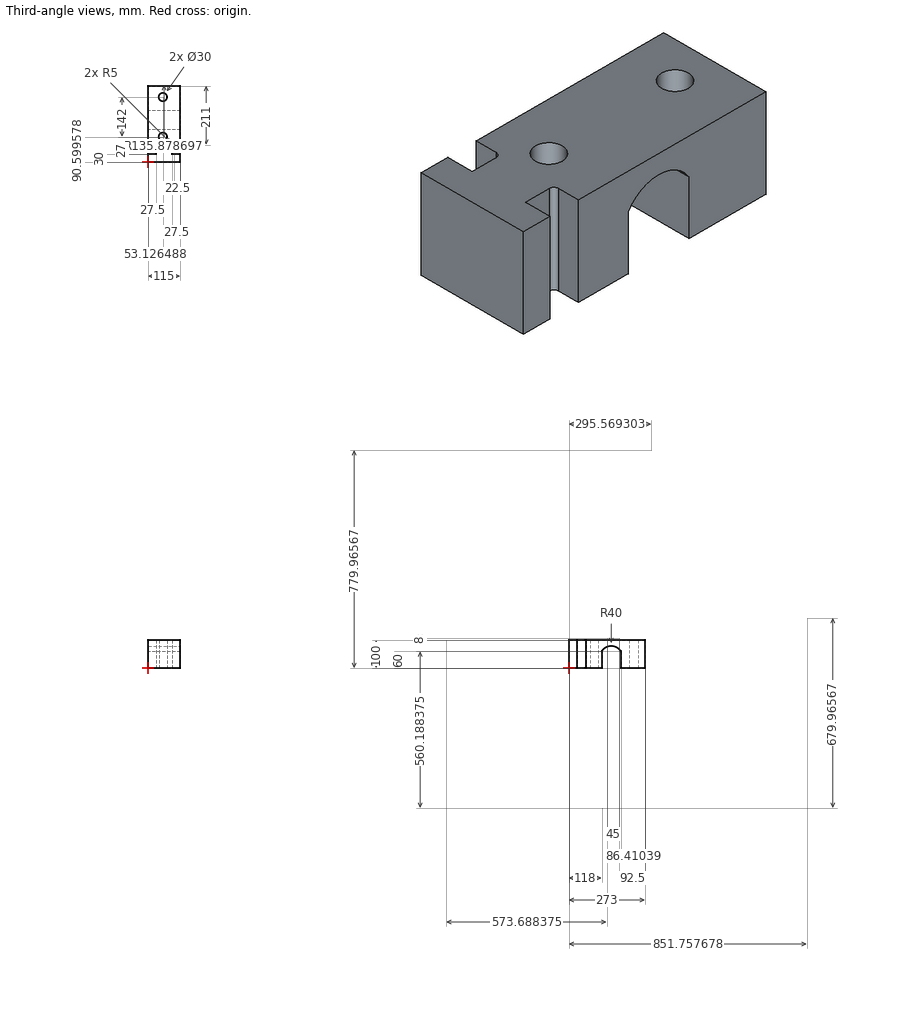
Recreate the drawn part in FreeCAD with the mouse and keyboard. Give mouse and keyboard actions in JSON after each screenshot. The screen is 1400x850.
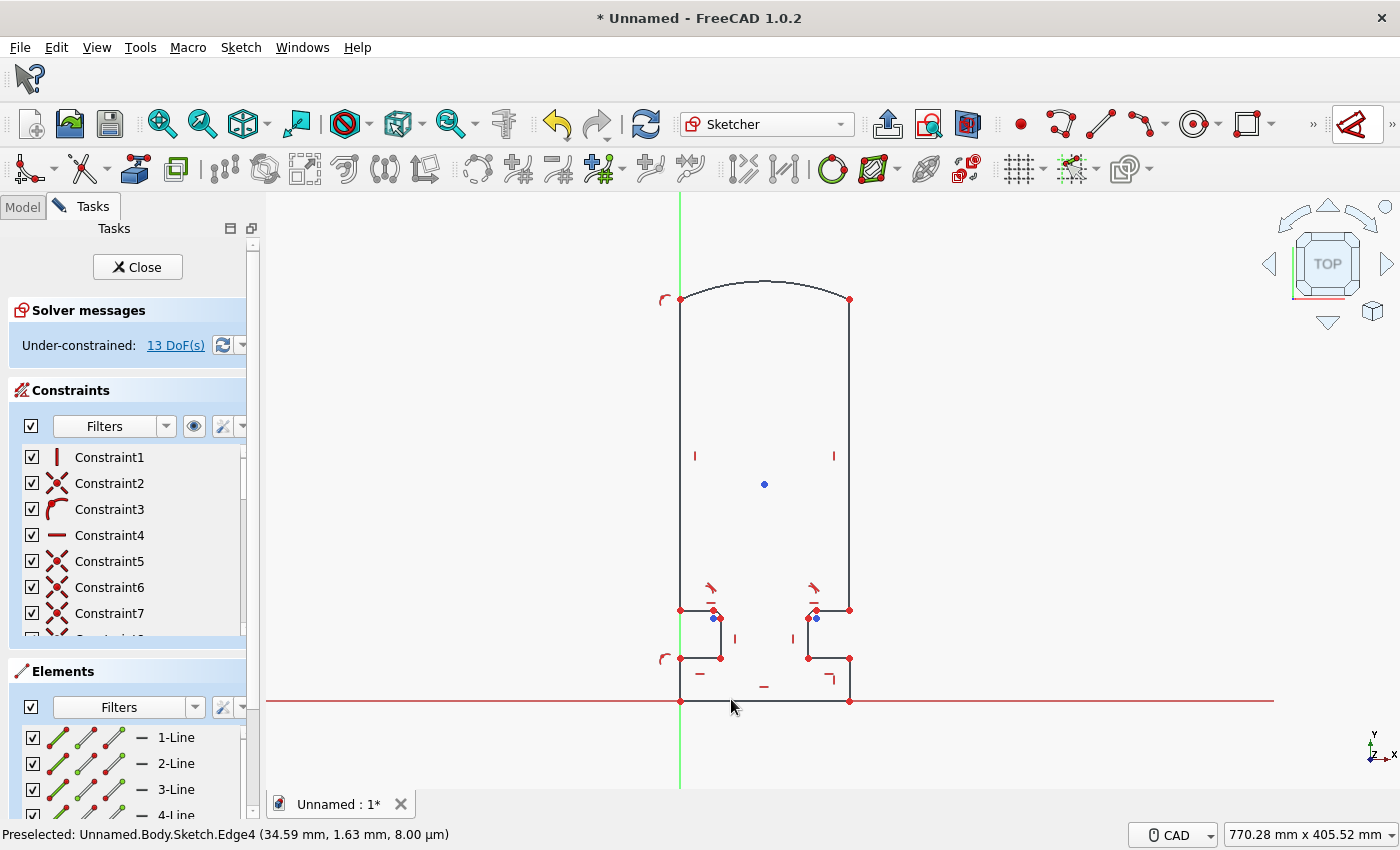
{"action": "scroll", "coordinate": [813, 611], "scroll_direction": "up", "scroll_amount": 7}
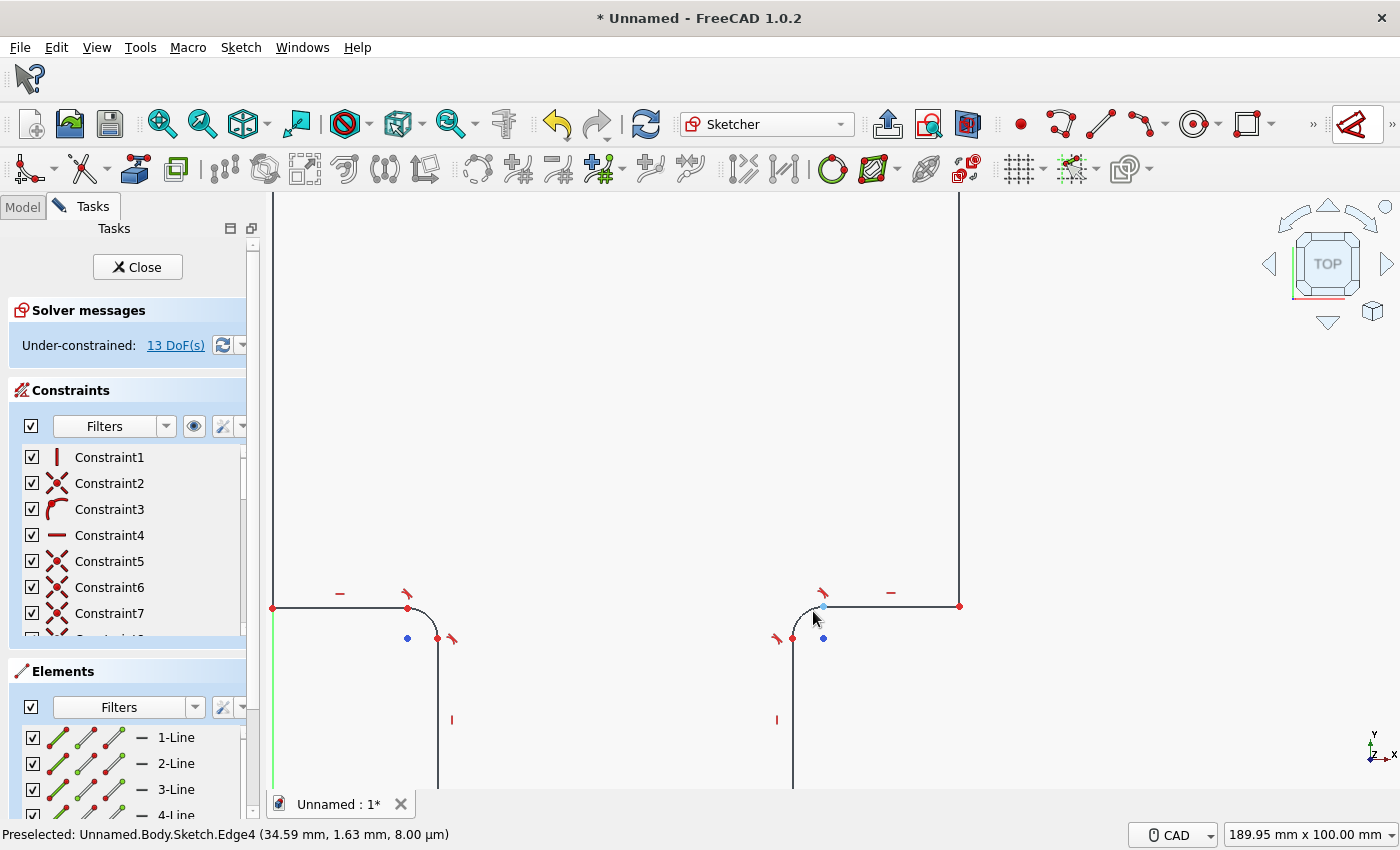
{"action": "left_click", "coordinate": [810, 610]}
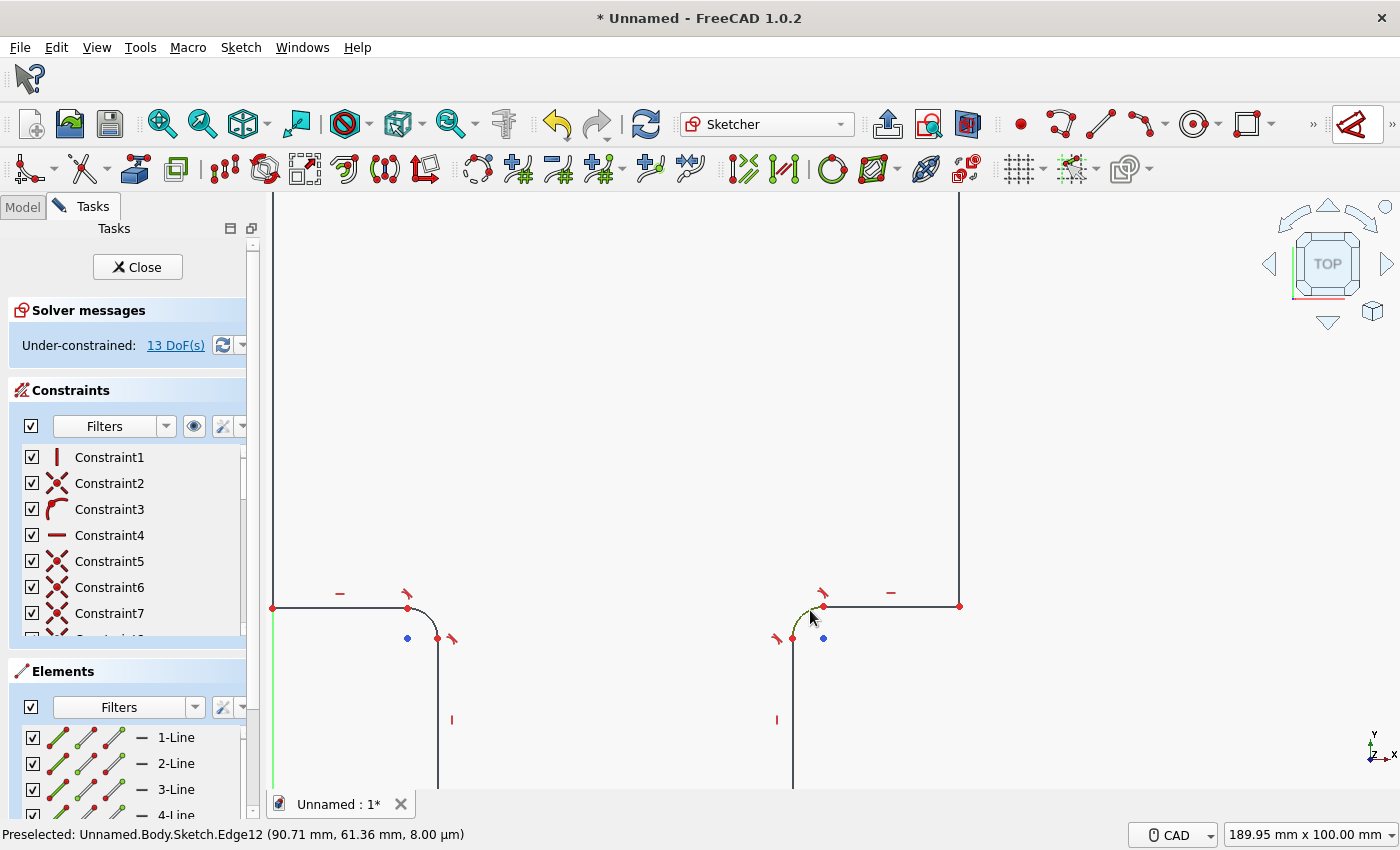
{"action": "left_click", "coordinate": [434, 625]}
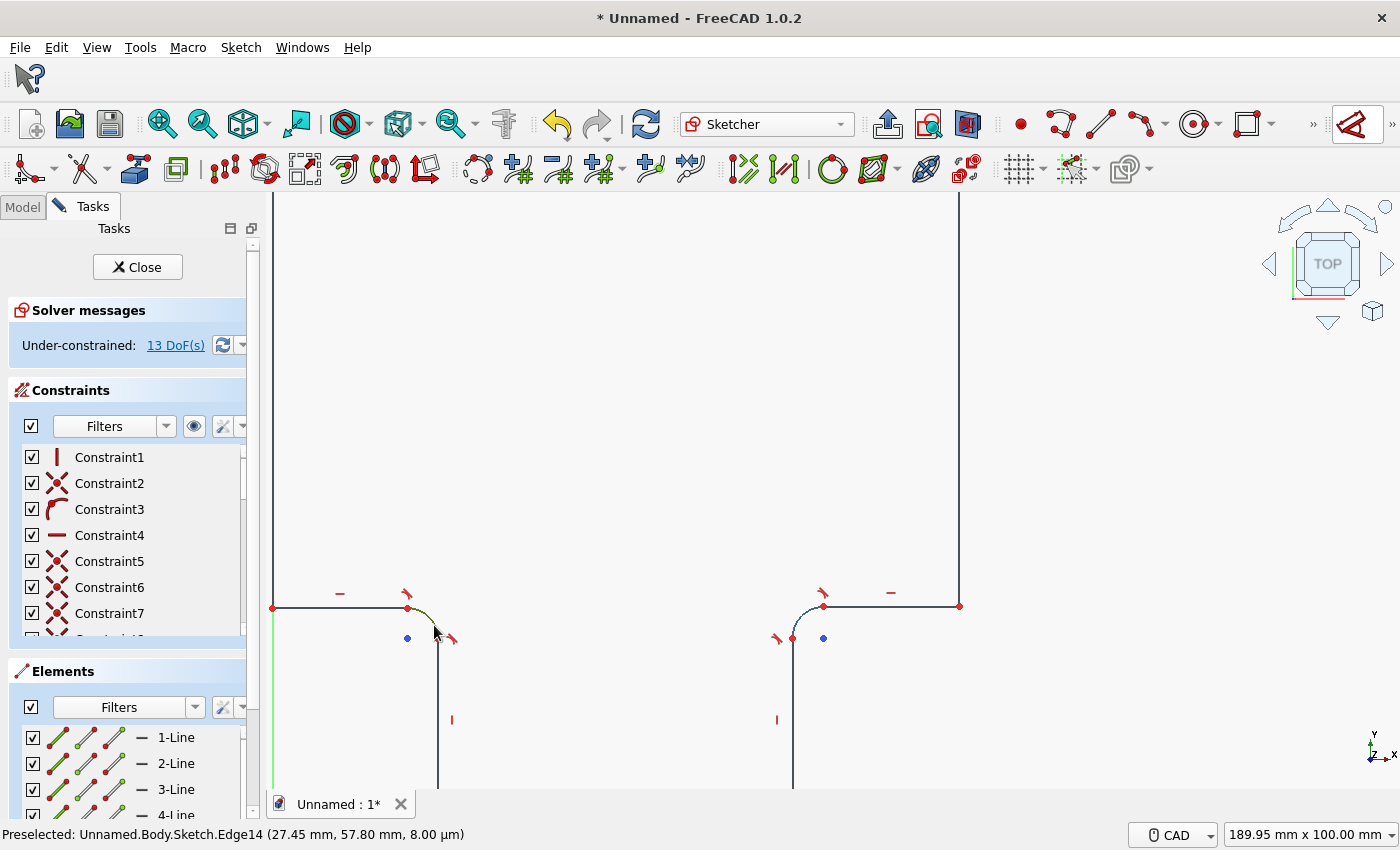
{"action": "key", "text": "e"}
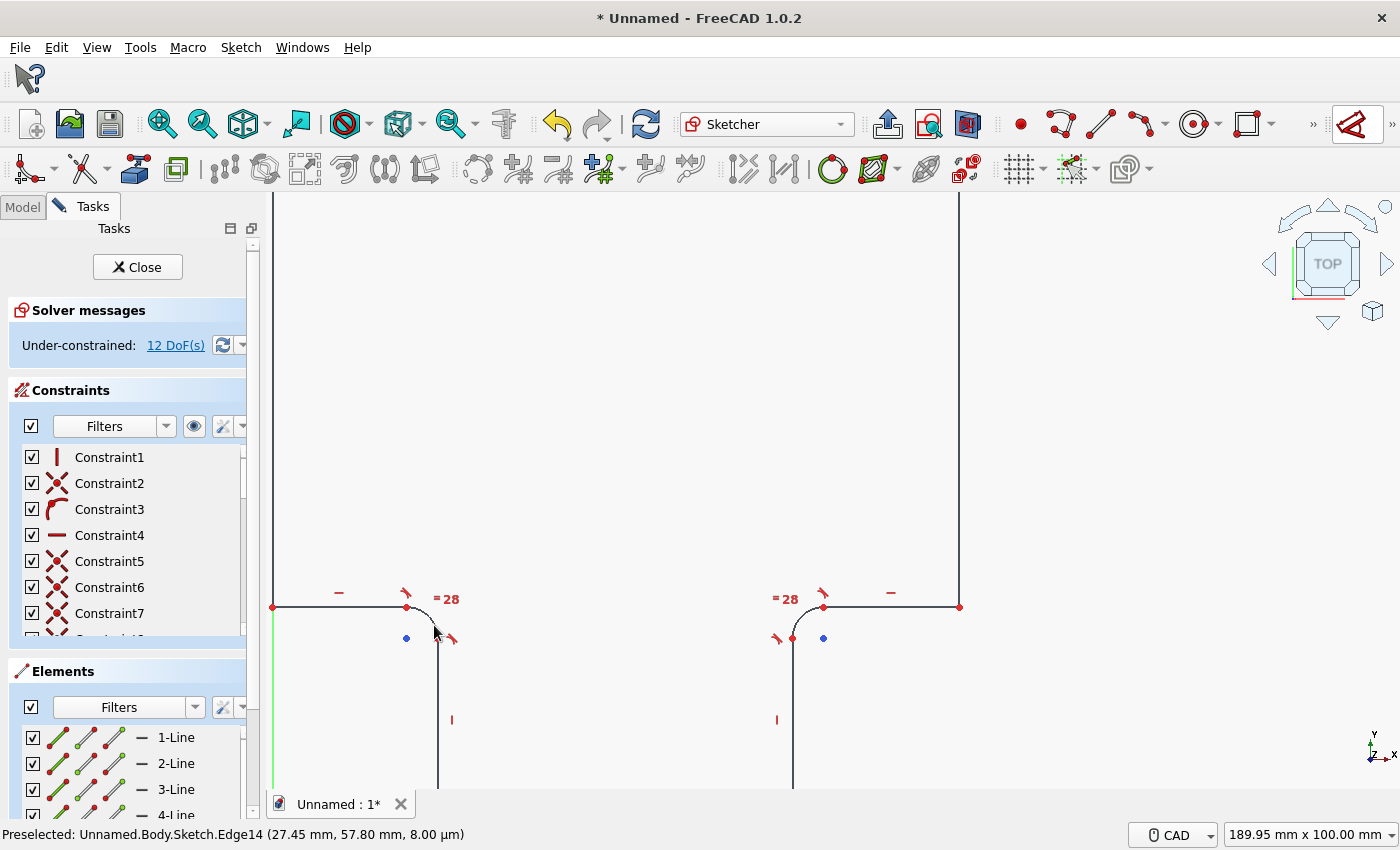
{"action": "key", "text": "d"}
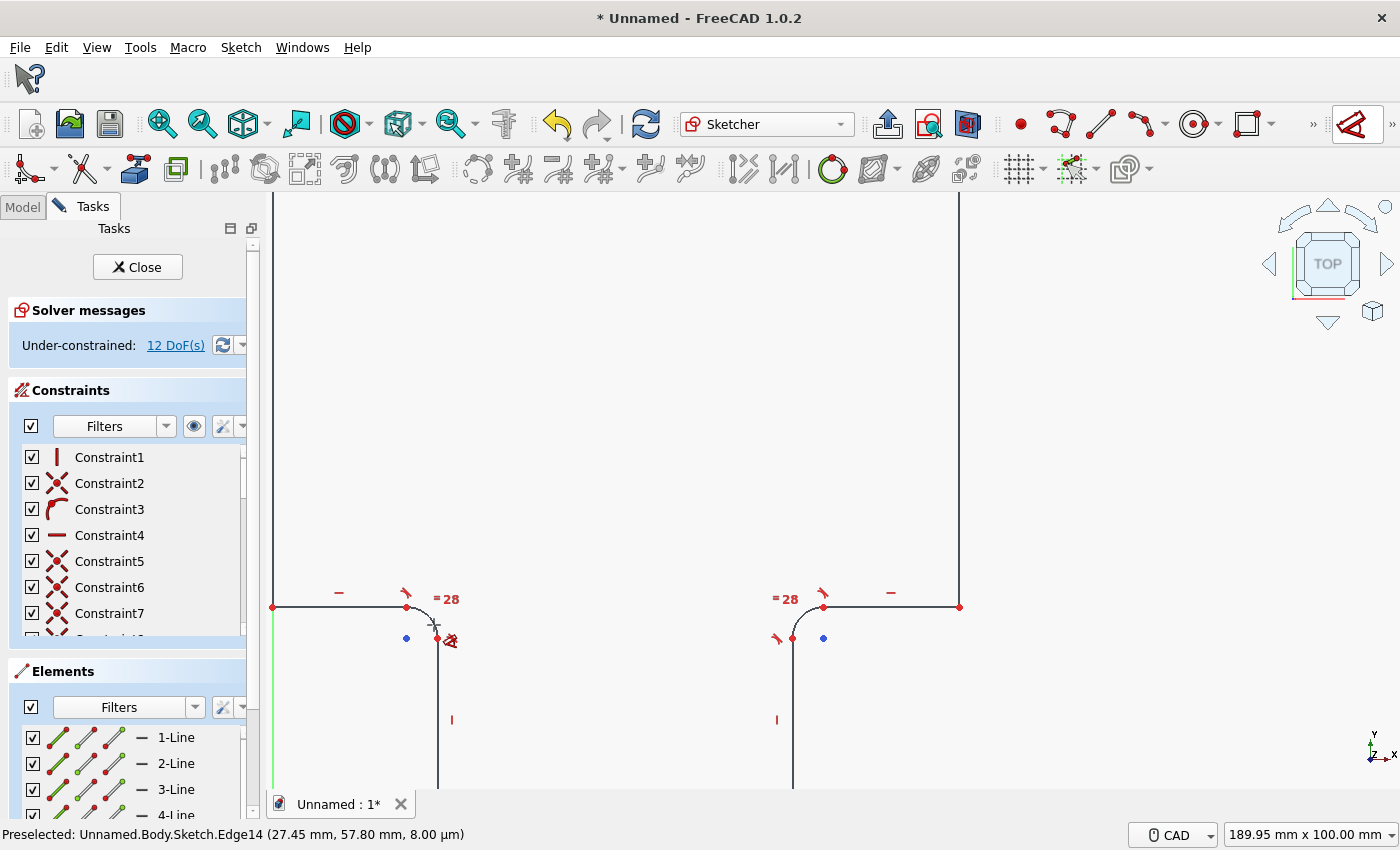
{"action": "scroll", "coordinate": [810, 611], "scroll_direction": "up", "scroll_amount": 2}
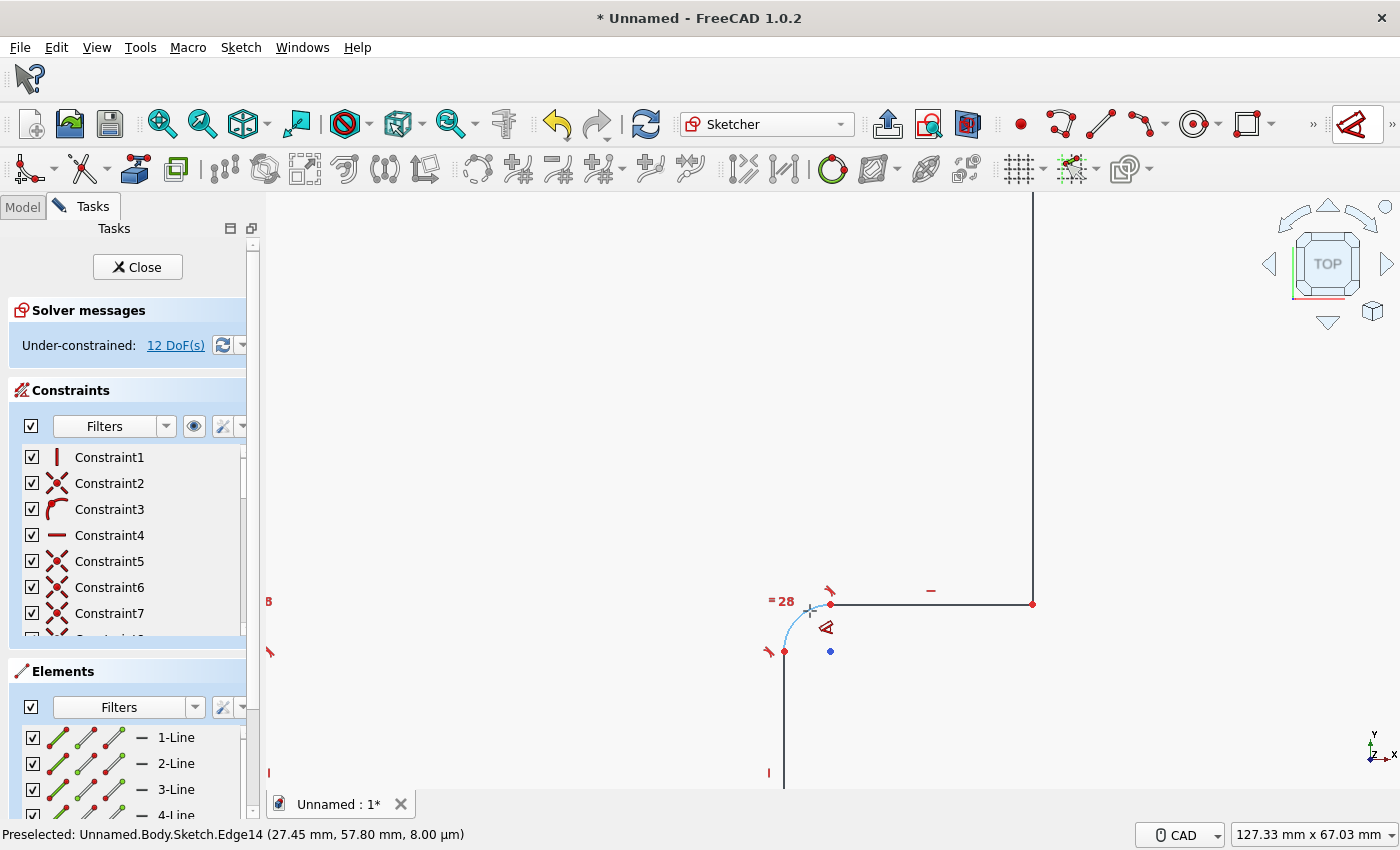
{"action": "left_click", "coordinate": [809, 610]}
{"action": "left_click", "coordinate": [794, 582]}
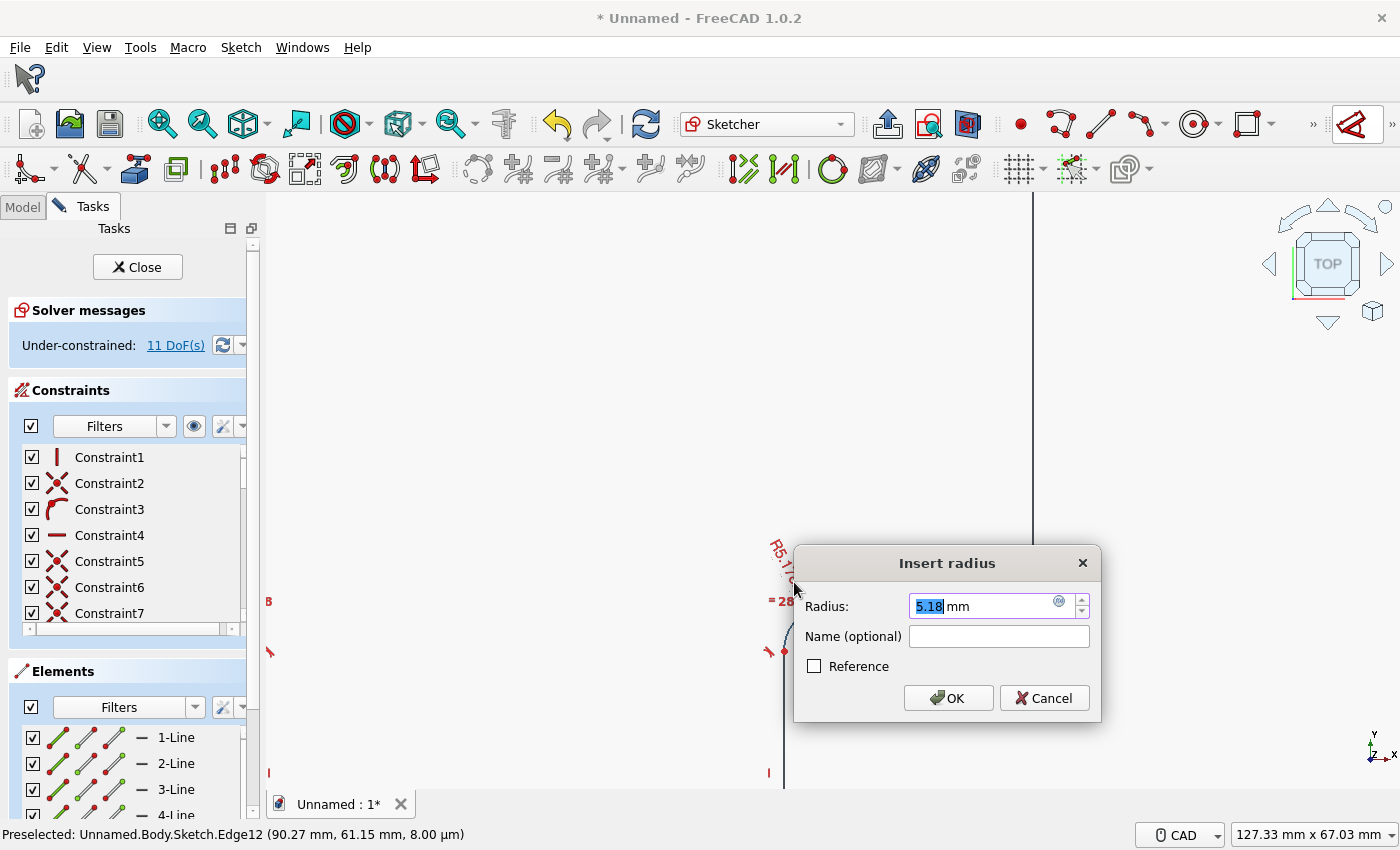
{"action": "type", "text": "5"}
{"action": "key", "text": "Return"}